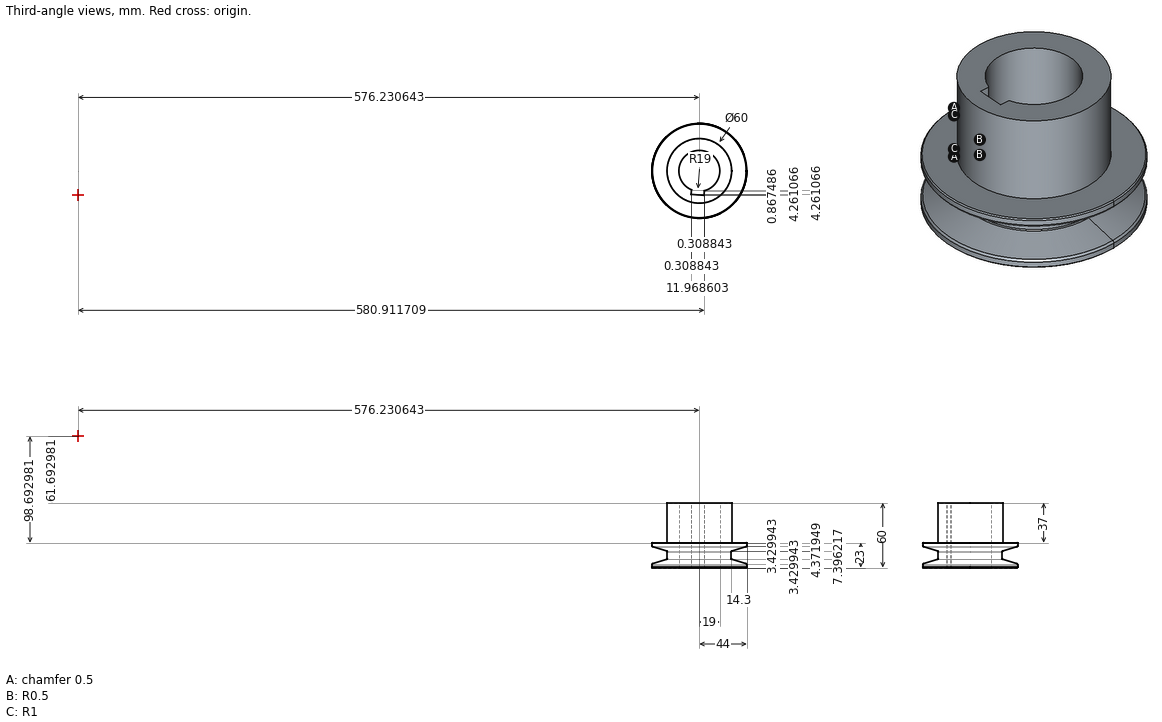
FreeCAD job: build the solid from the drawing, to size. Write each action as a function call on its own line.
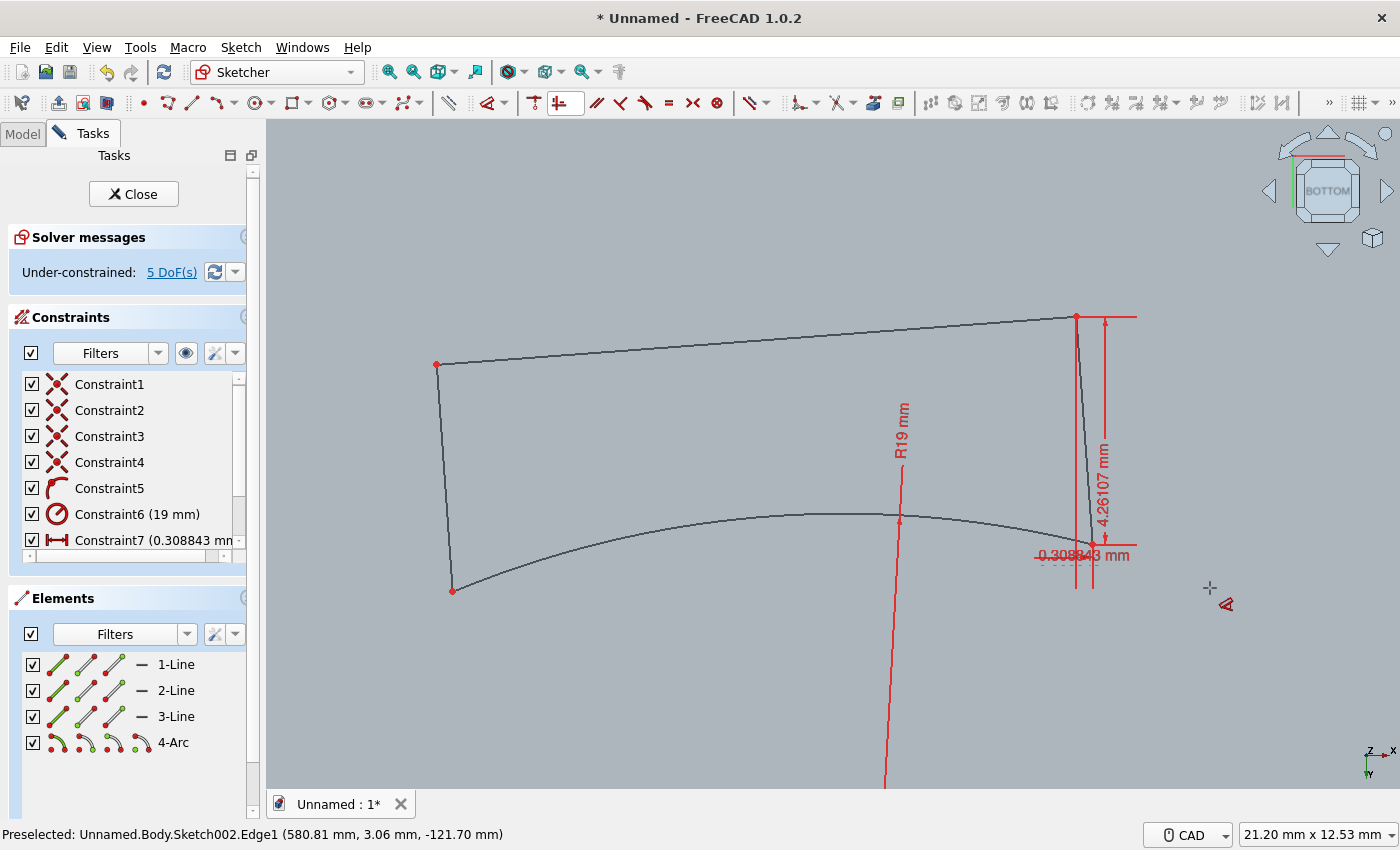
click(884, 331)
click(403, 341)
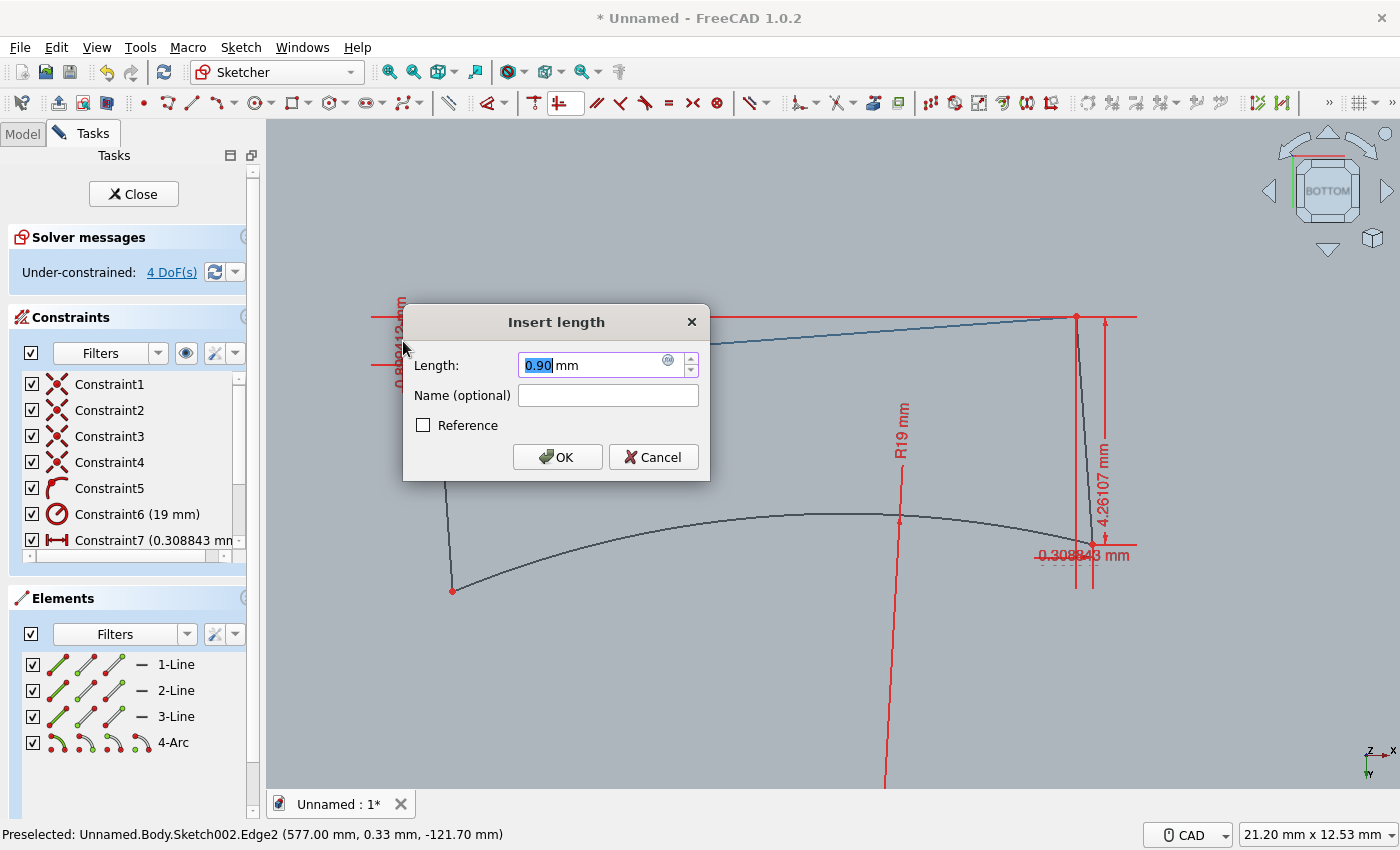
text(0.867486)
key(Return)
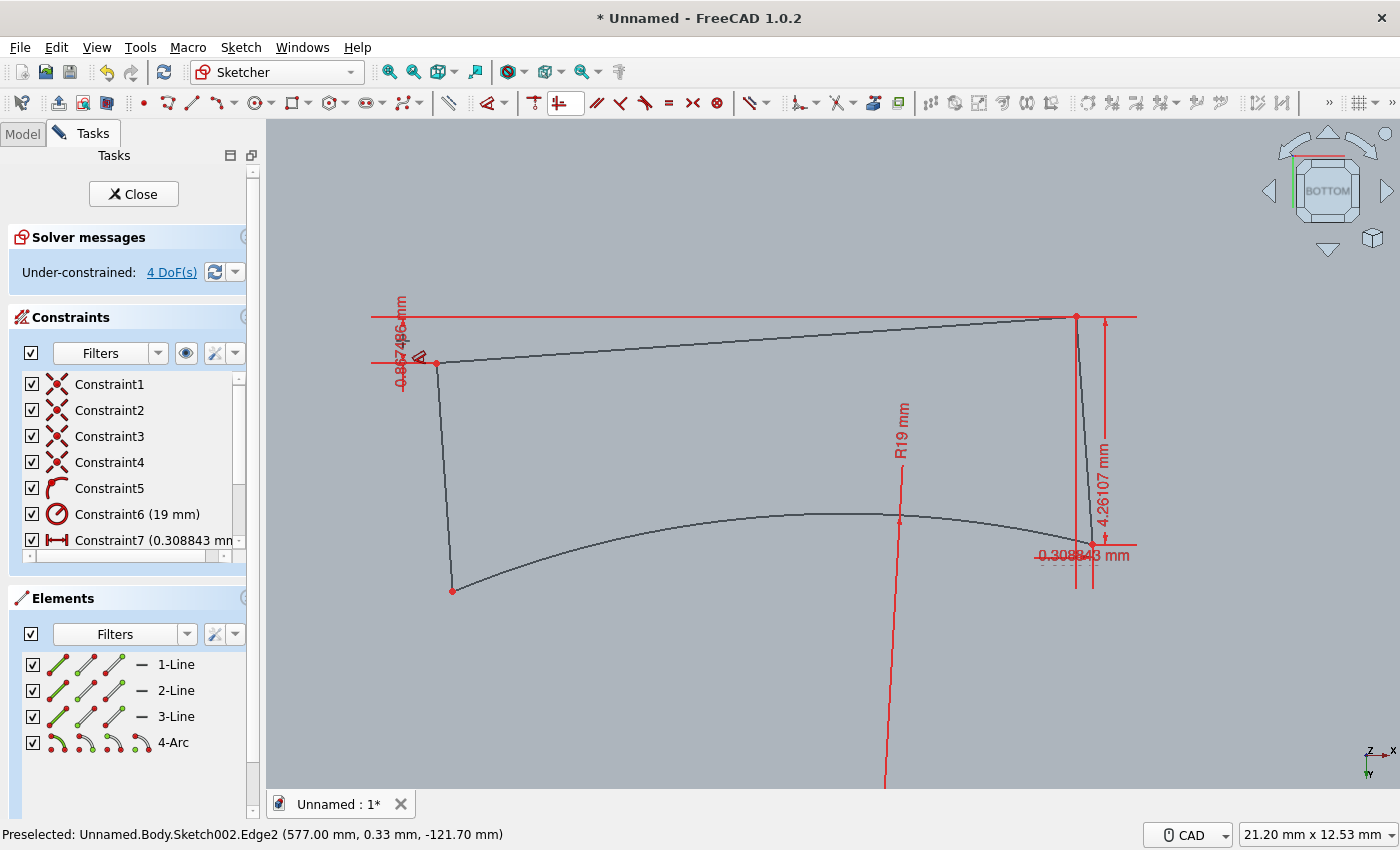
scroll(442, 432, up, 5)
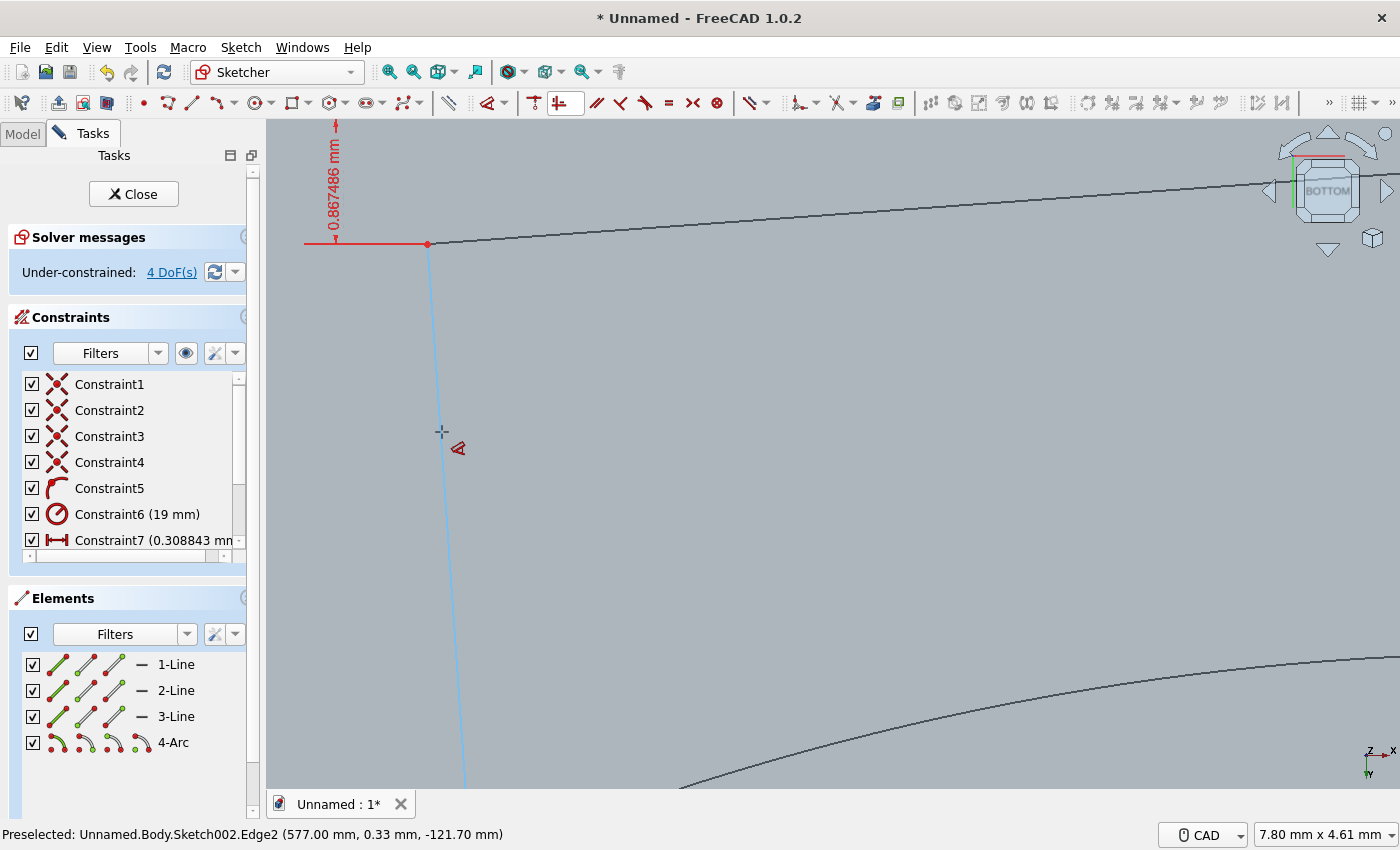
click(441, 431)
click(449, 210)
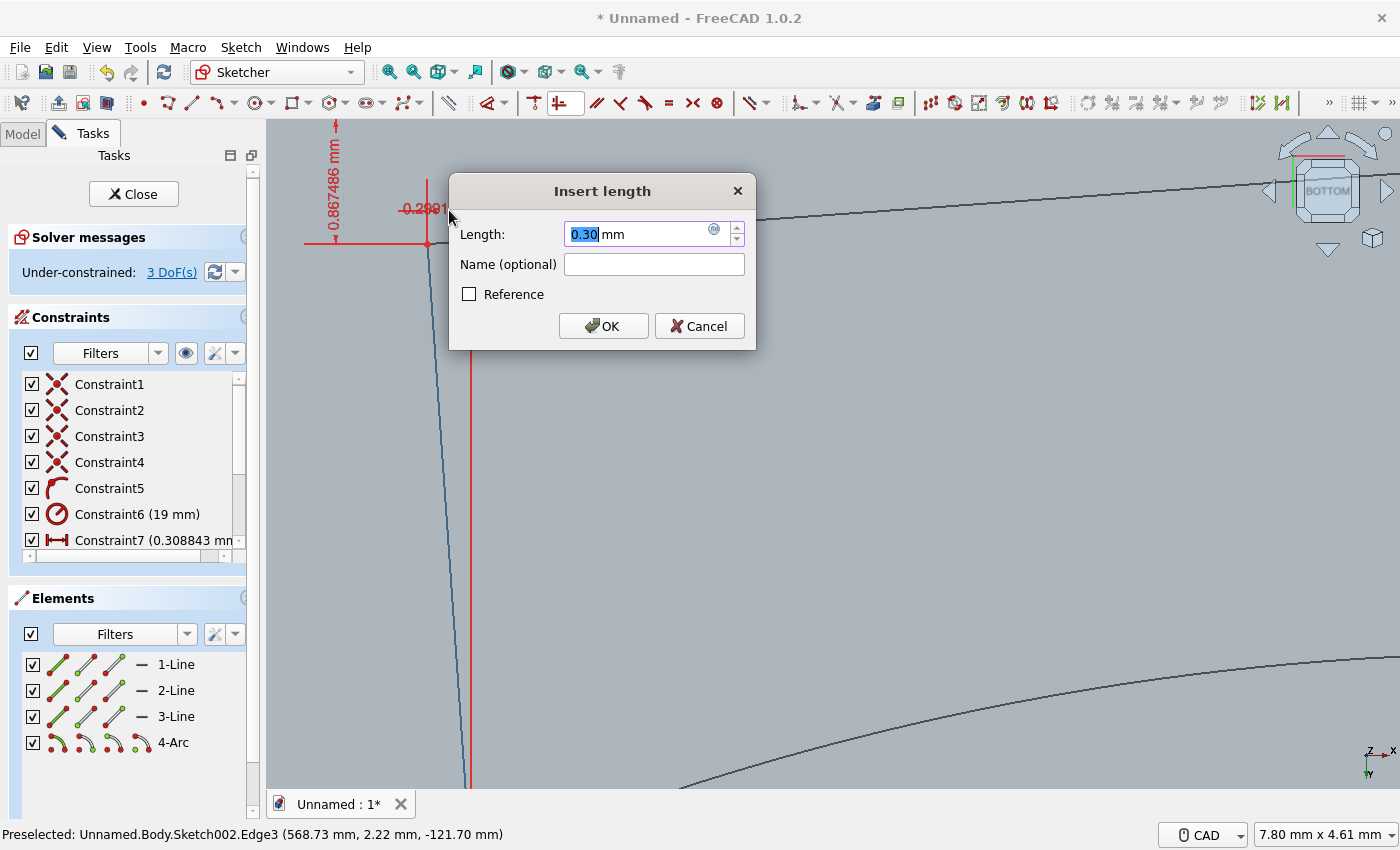
text(0.308843)
key(Return)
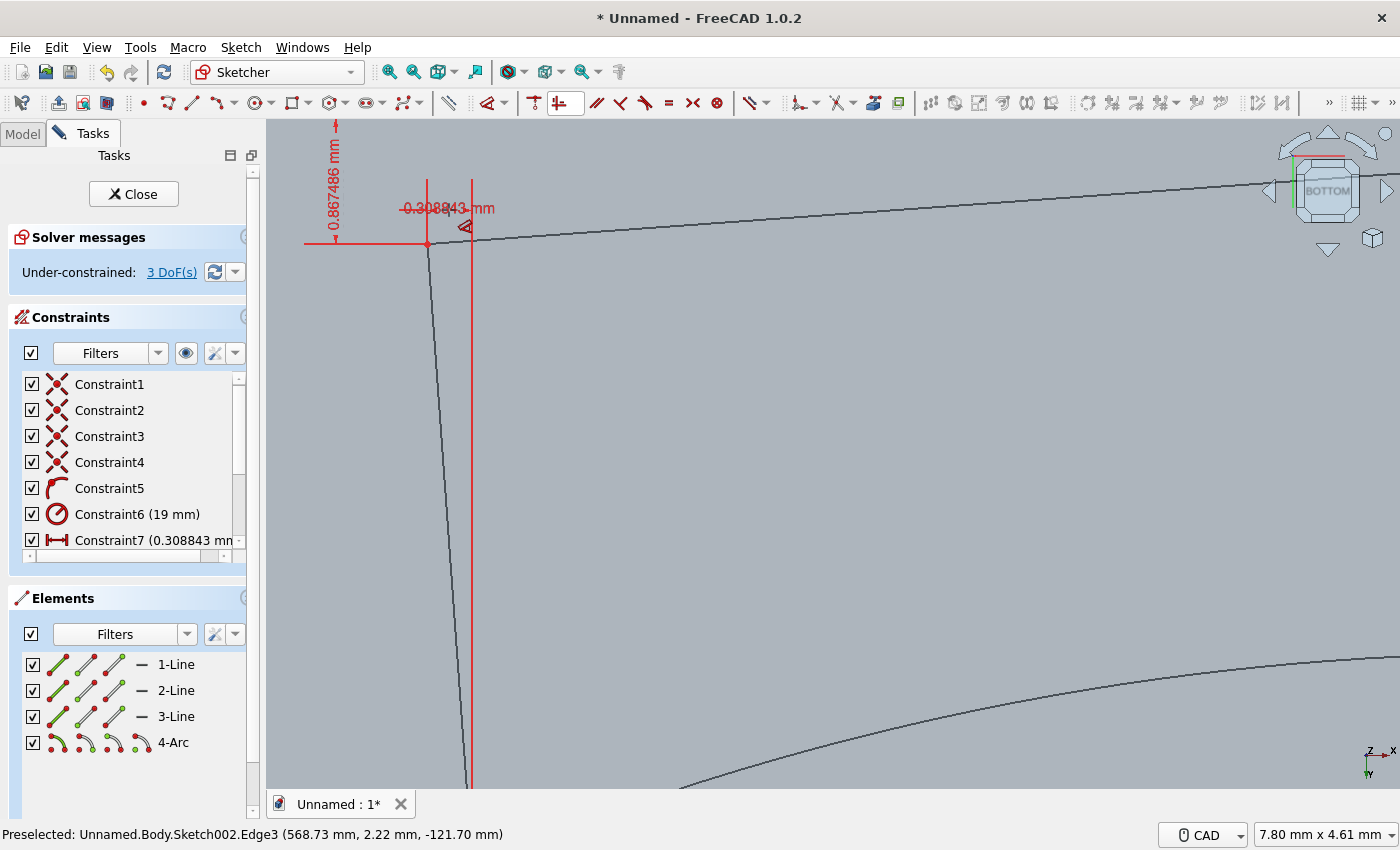
click(441, 431)
click(393, 503)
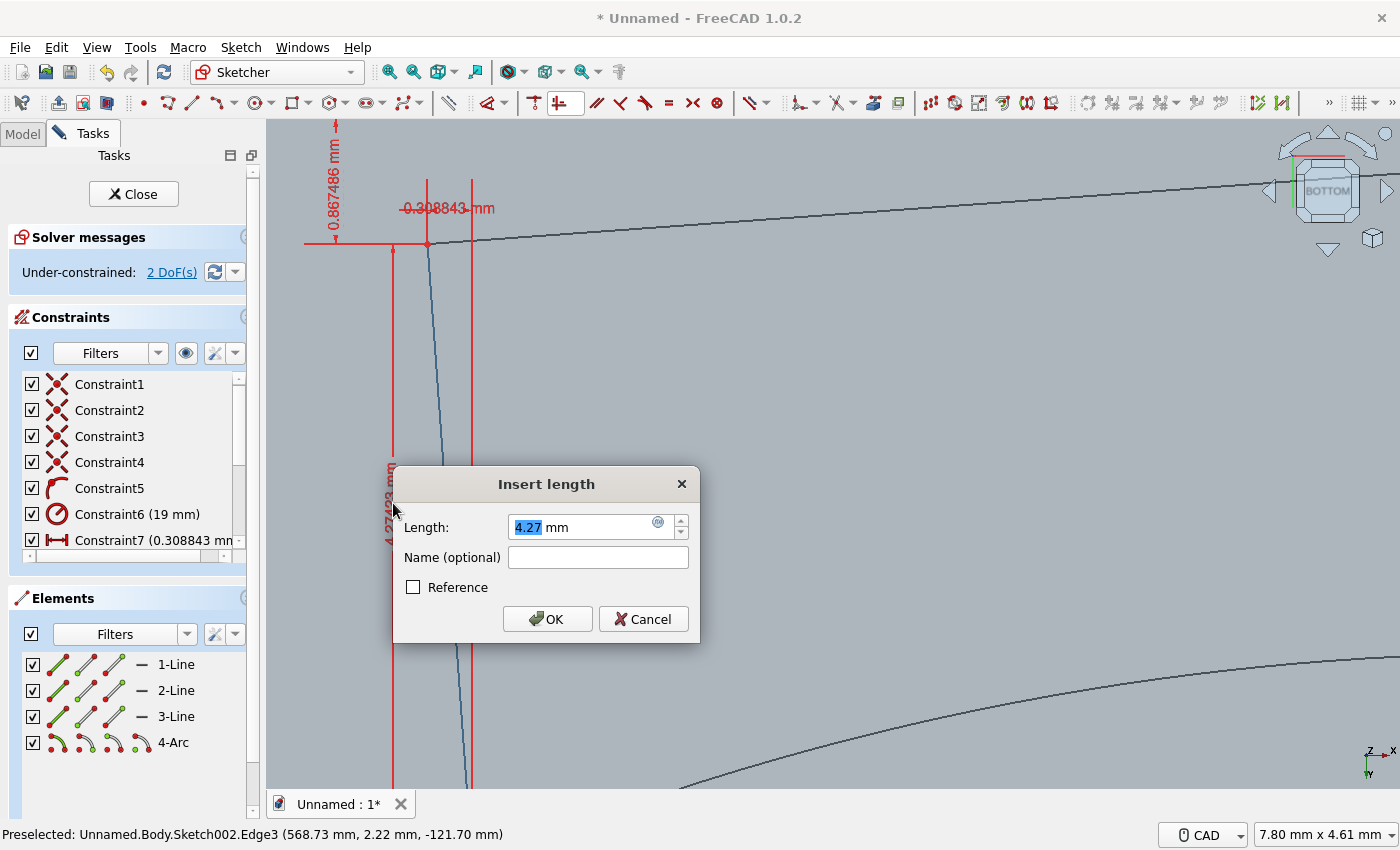
text(4.261066)
key(Return)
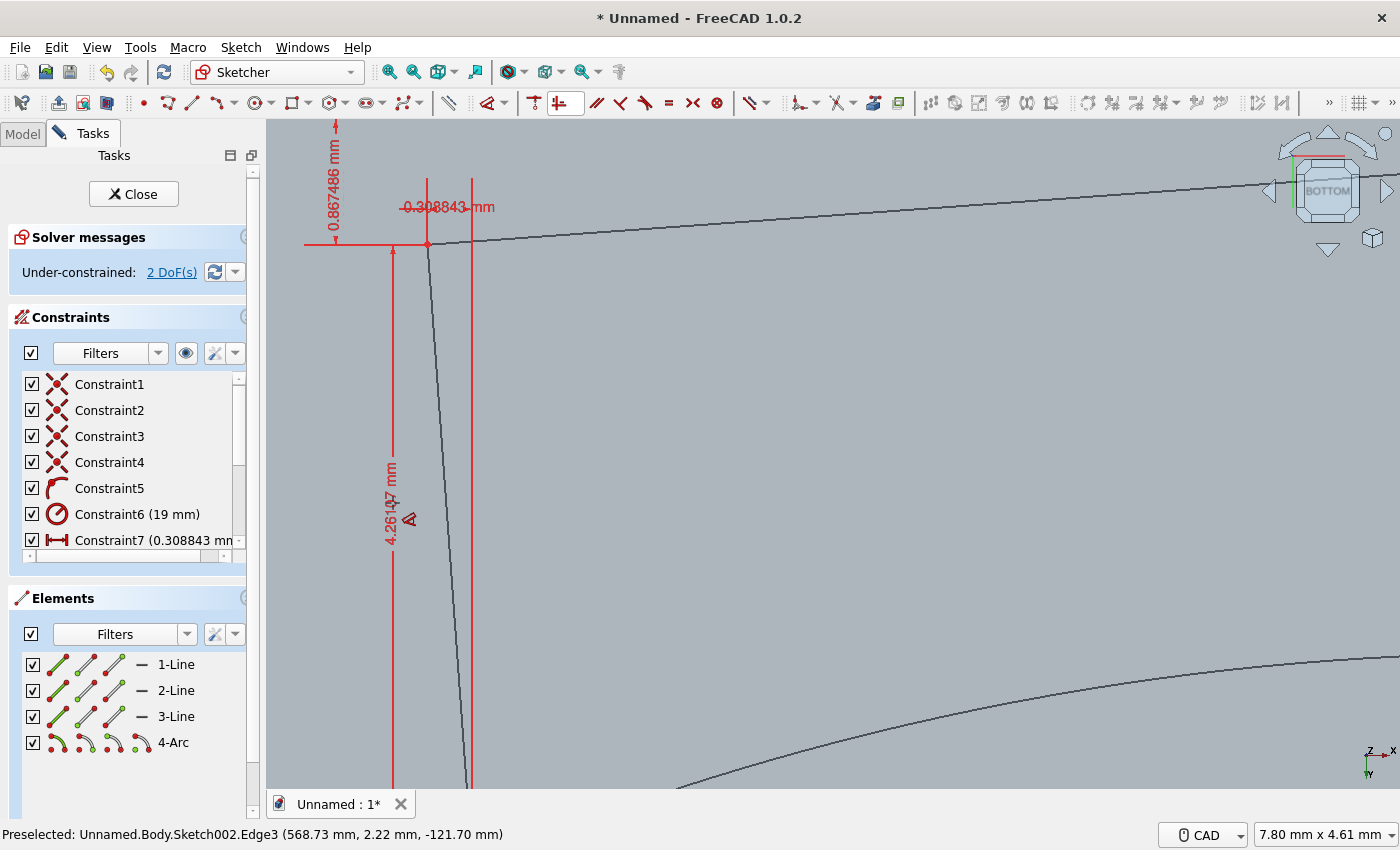
click(949, 207)
click(831, 279)